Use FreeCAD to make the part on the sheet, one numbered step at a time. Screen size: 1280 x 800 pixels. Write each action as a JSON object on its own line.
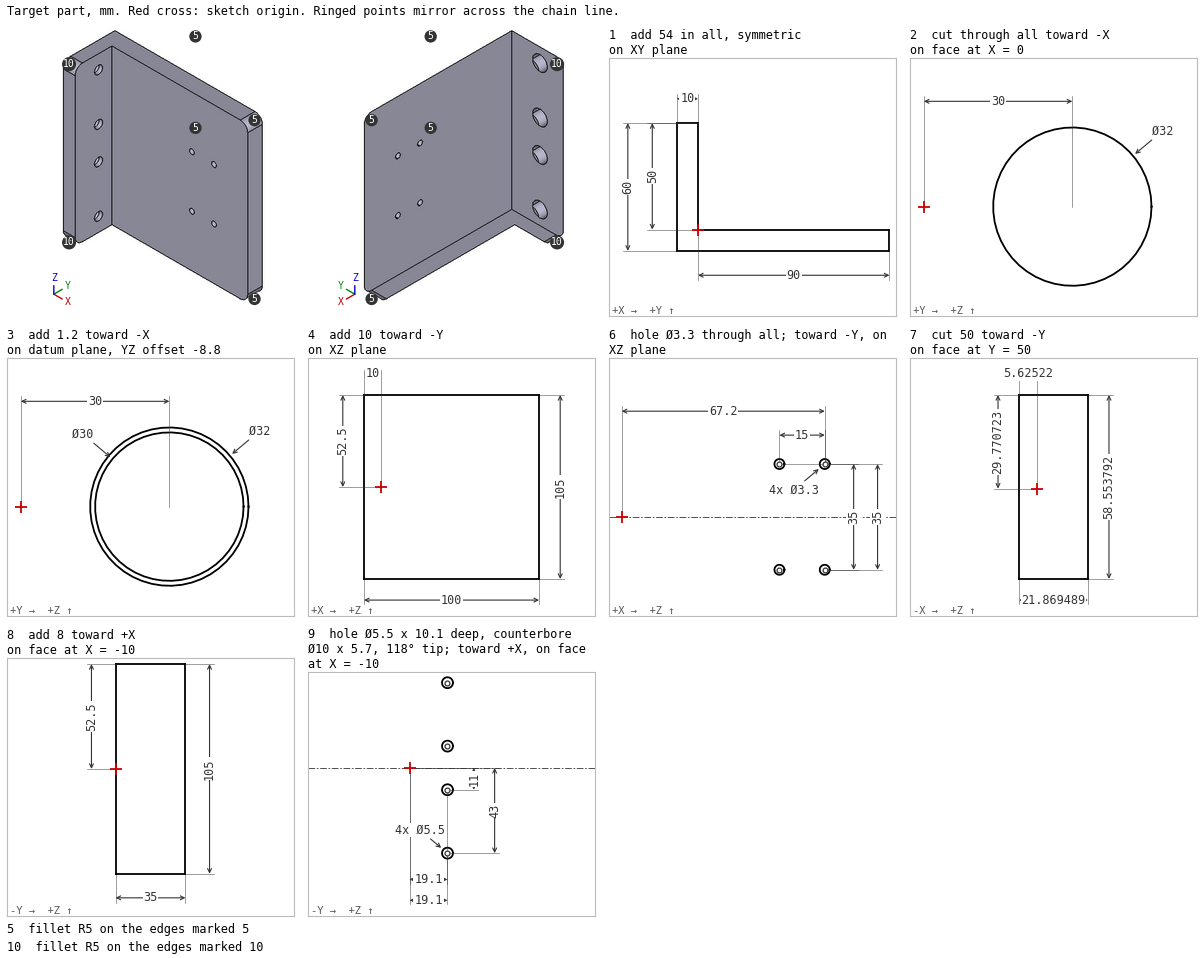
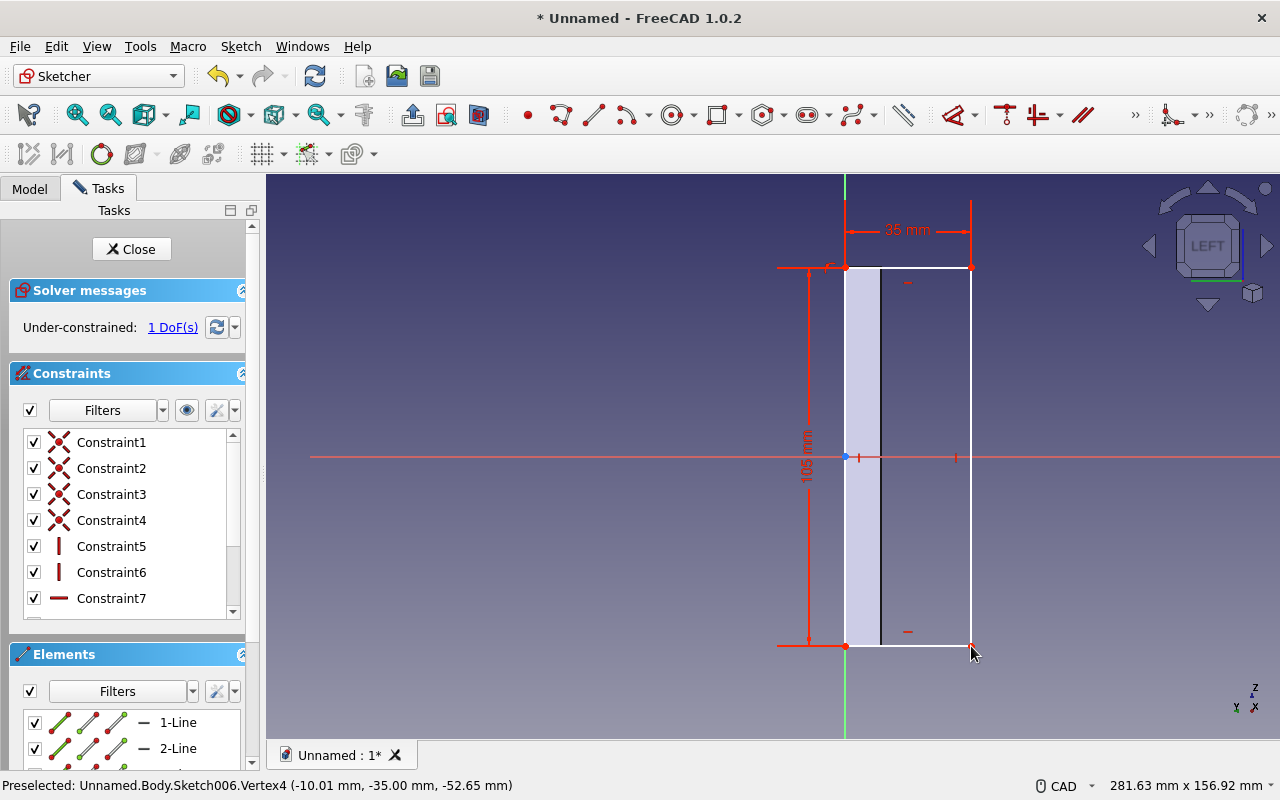
{"action": "left_click", "coordinate": [952, 116]}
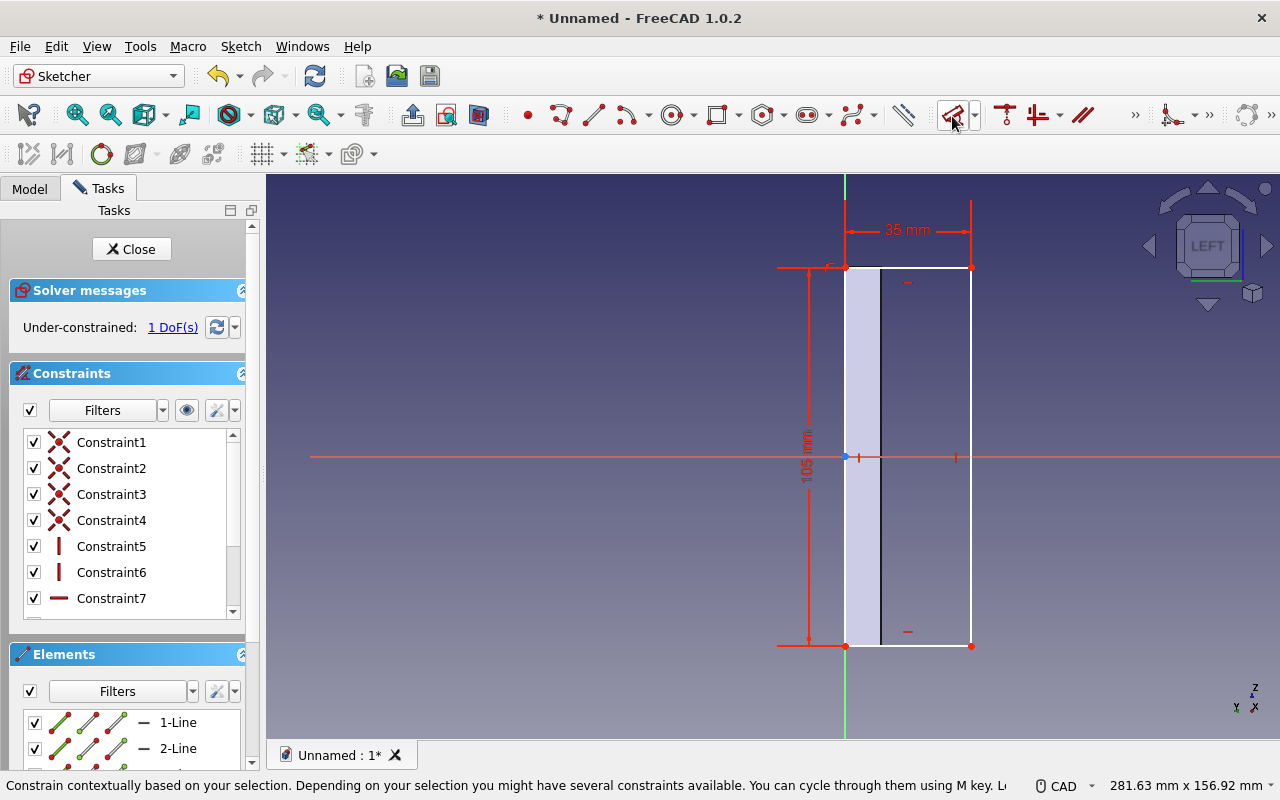
{"action": "left_click", "coordinate": [845, 268]}
{"action": "left_click", "coordinate": [811, 362]}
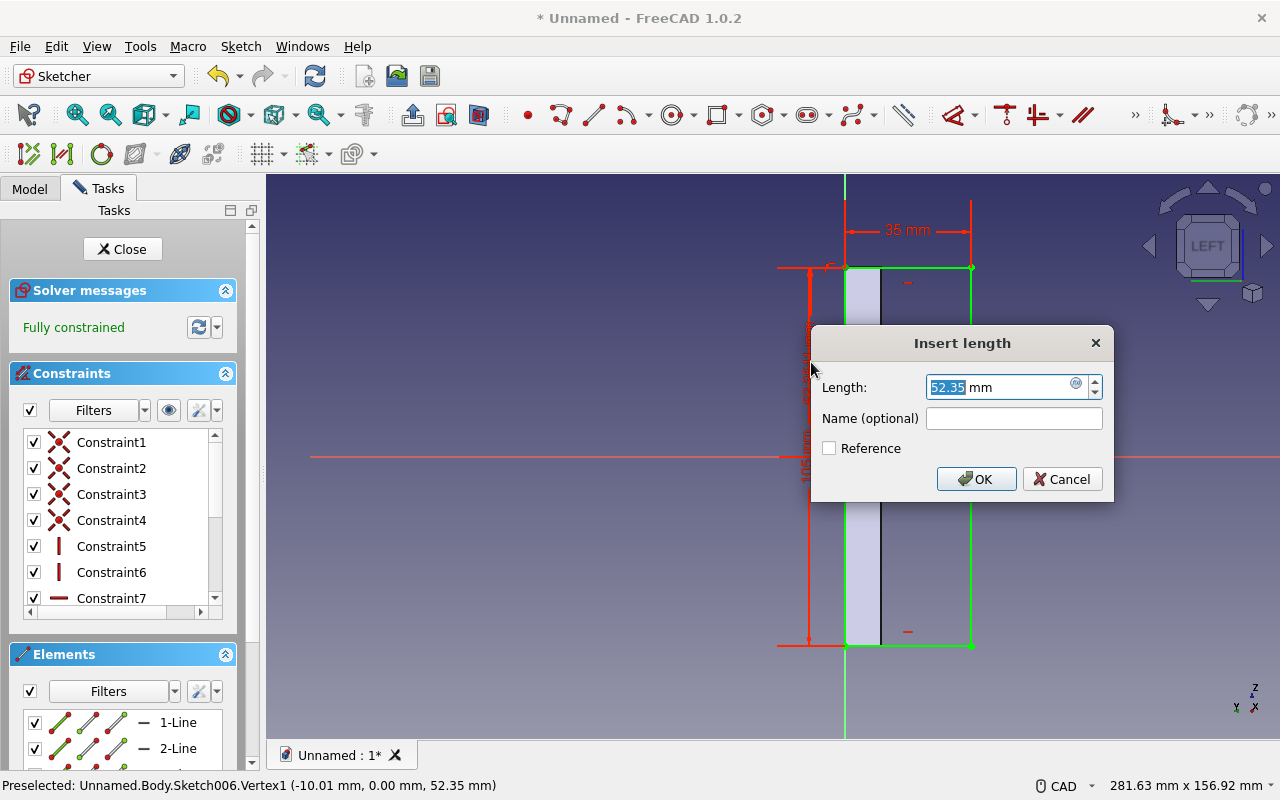
{"action": "type", "text": "52.5"}
{"action": "key", "text": "Return"}
{"action": "key", "text": "Escape"}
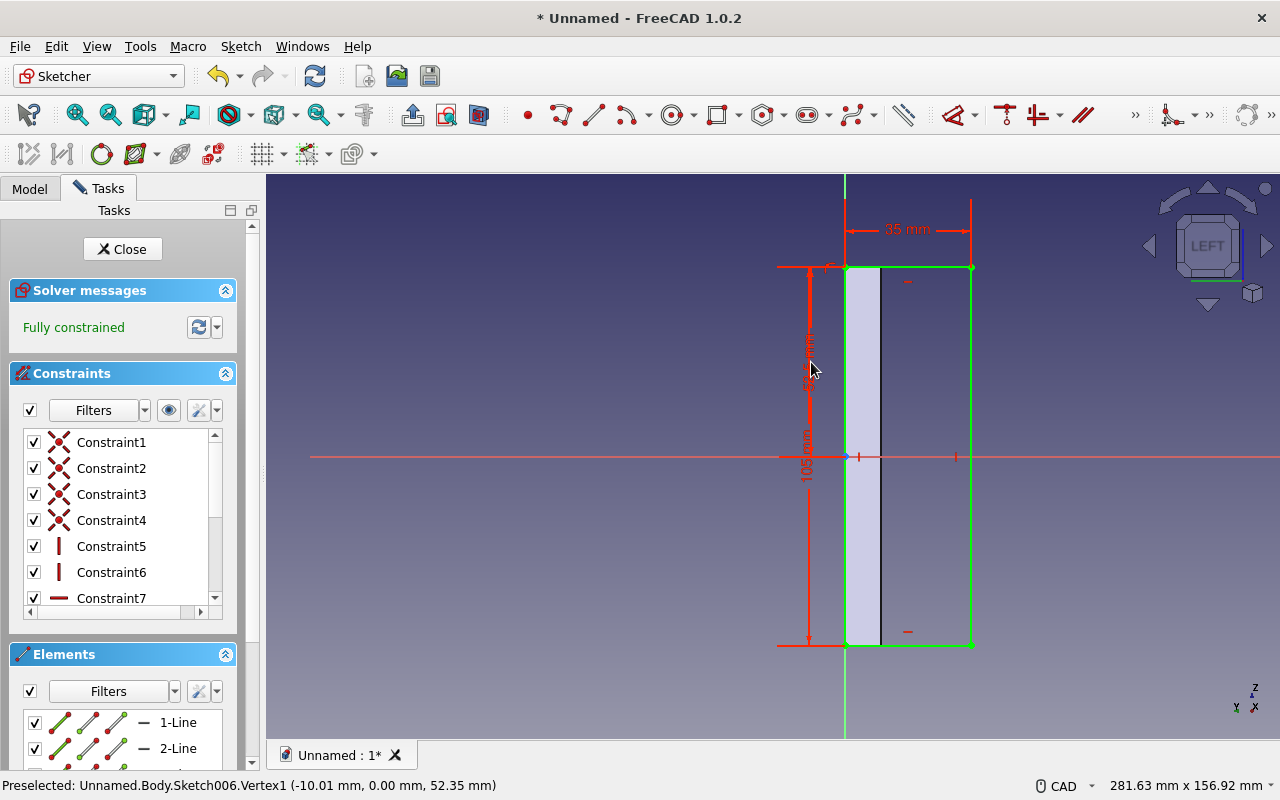
{"action": "left_click", "coordinate": [123, 249]}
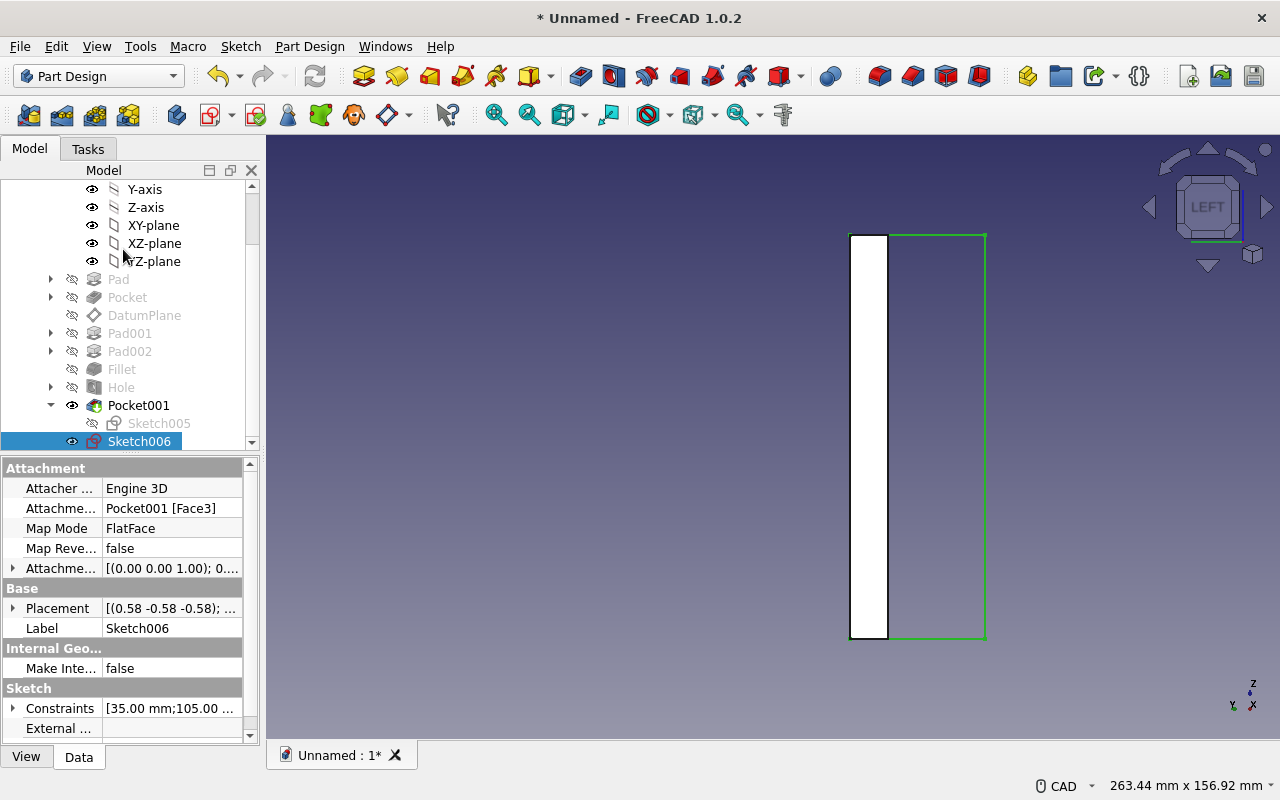
{"action": "left_click", "coordinate": [364, 76]}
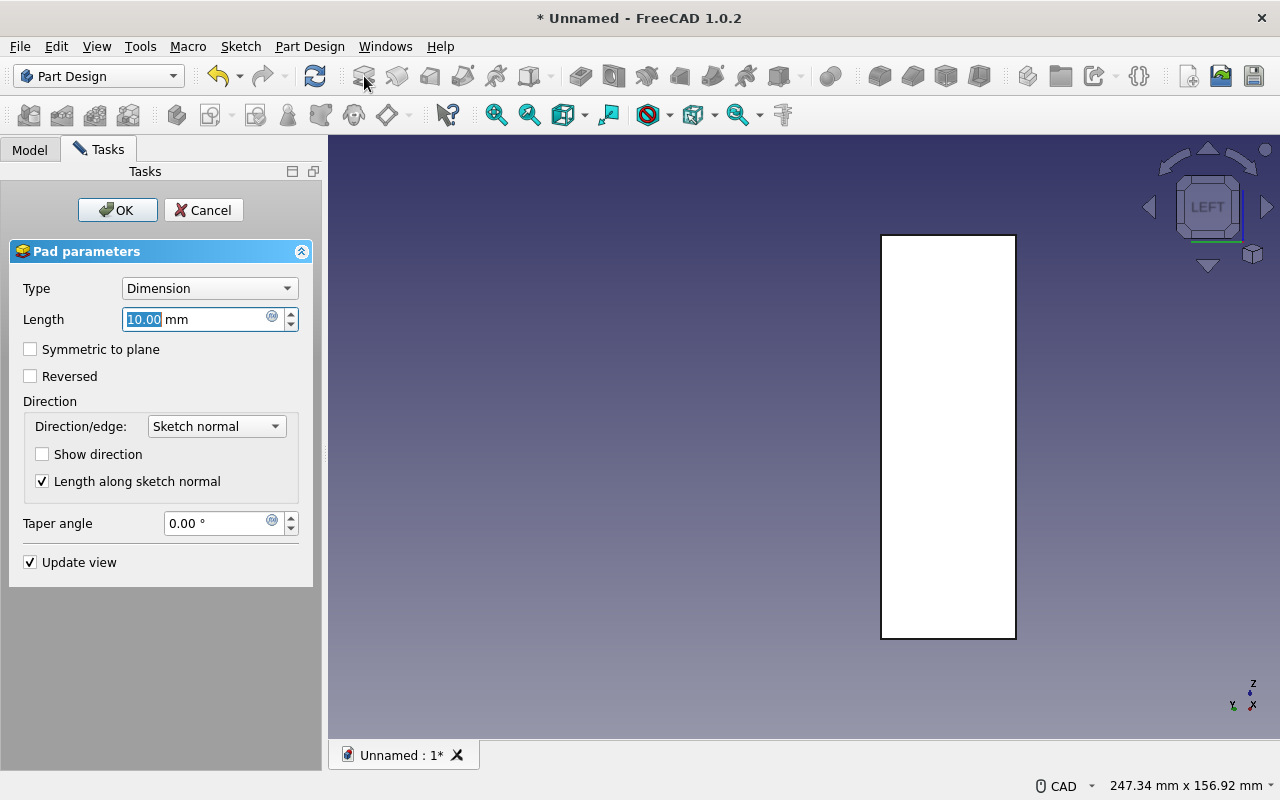
{"action": "type", "text": "8"}
{"action": "key", "text": "Tab"}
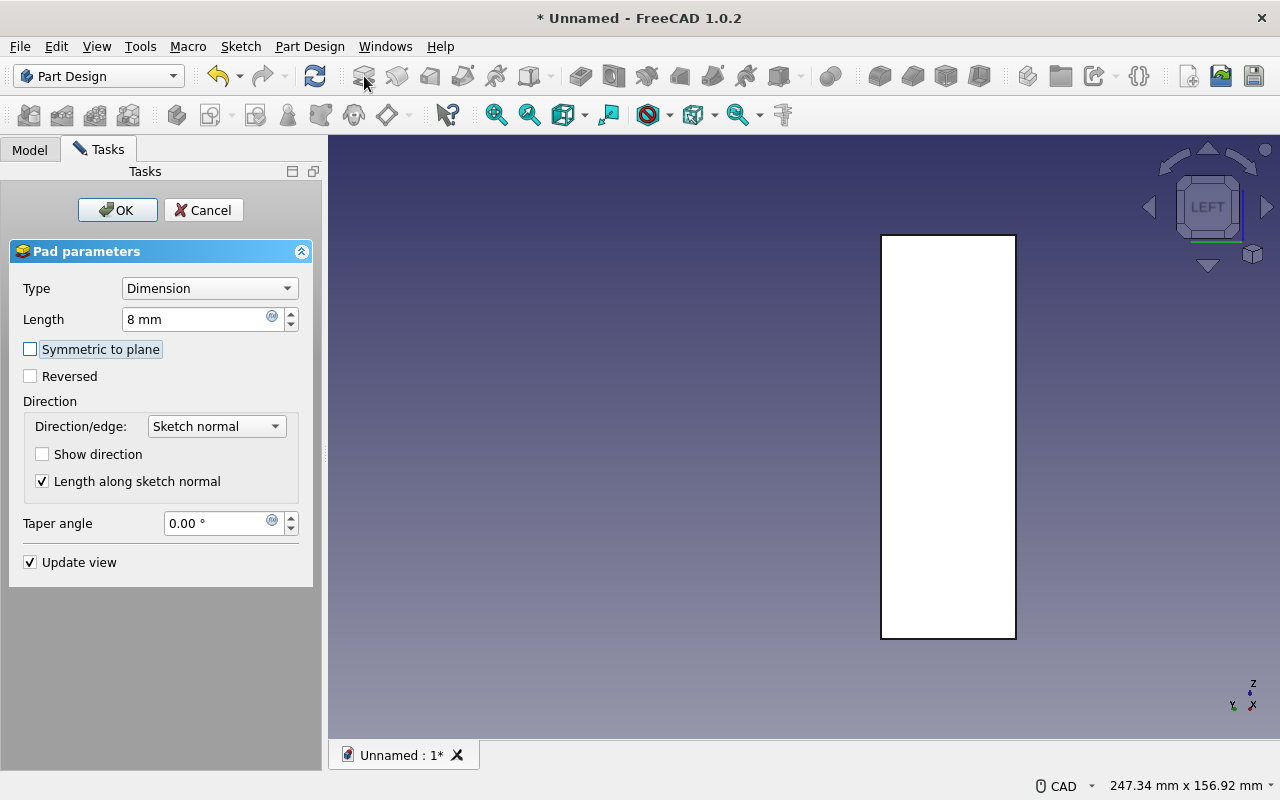
{"action": "left_click", "coordinate": [31, 376]}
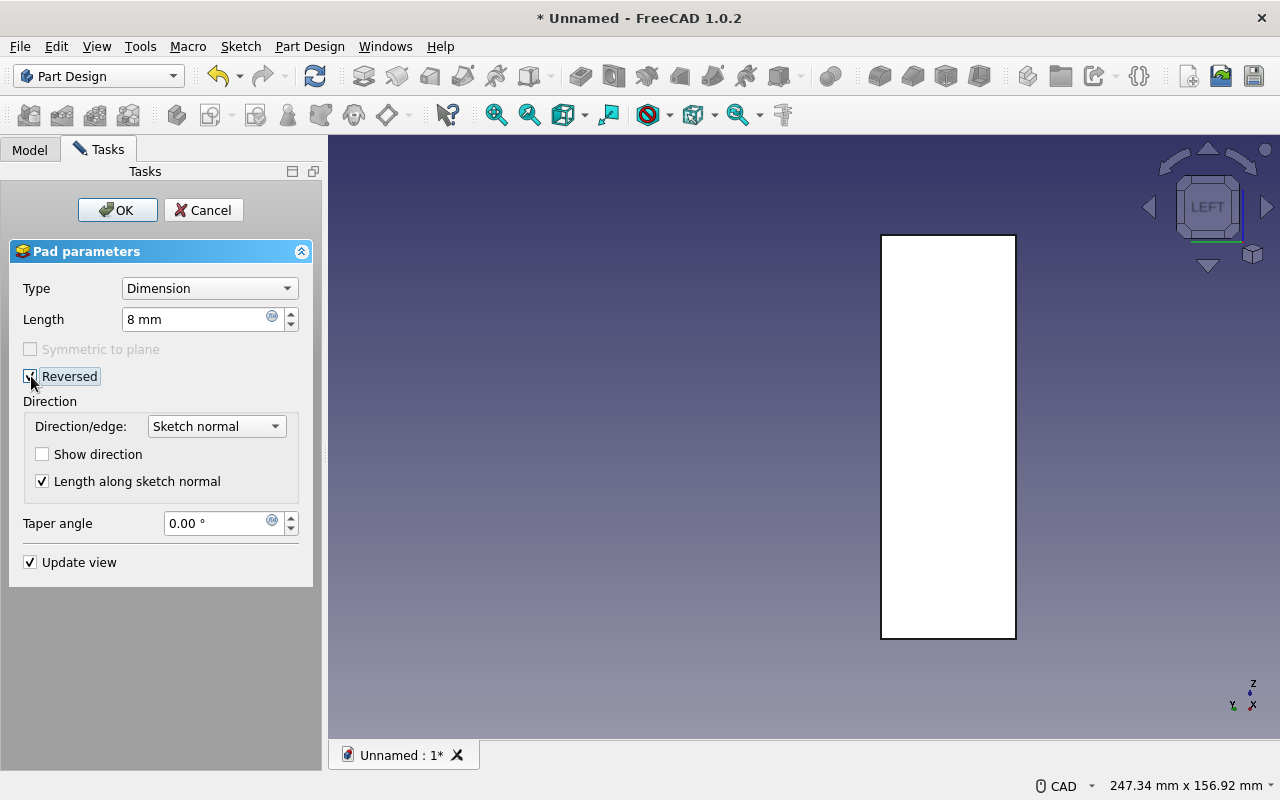
{"action": "left_click", "coordinate": [118, 210]}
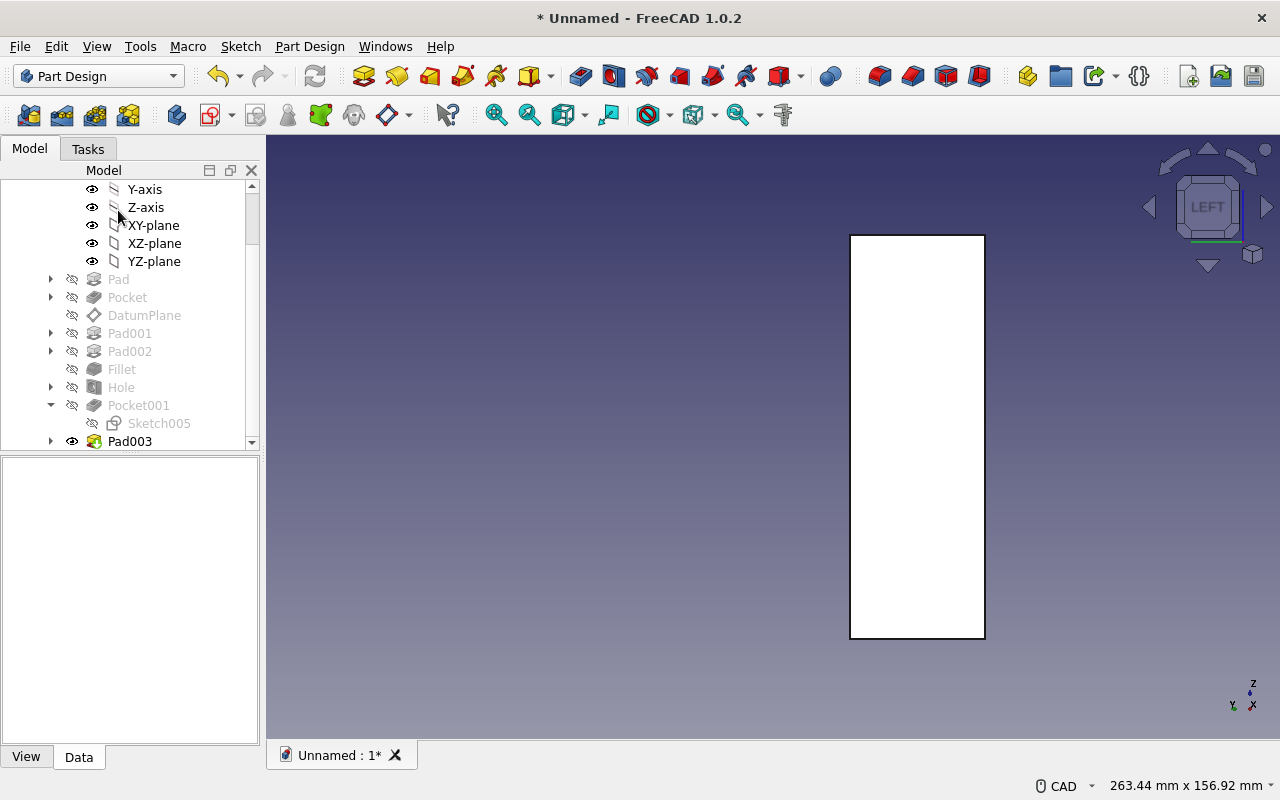
{"action": "left_click", "coordinate": [917, 321]}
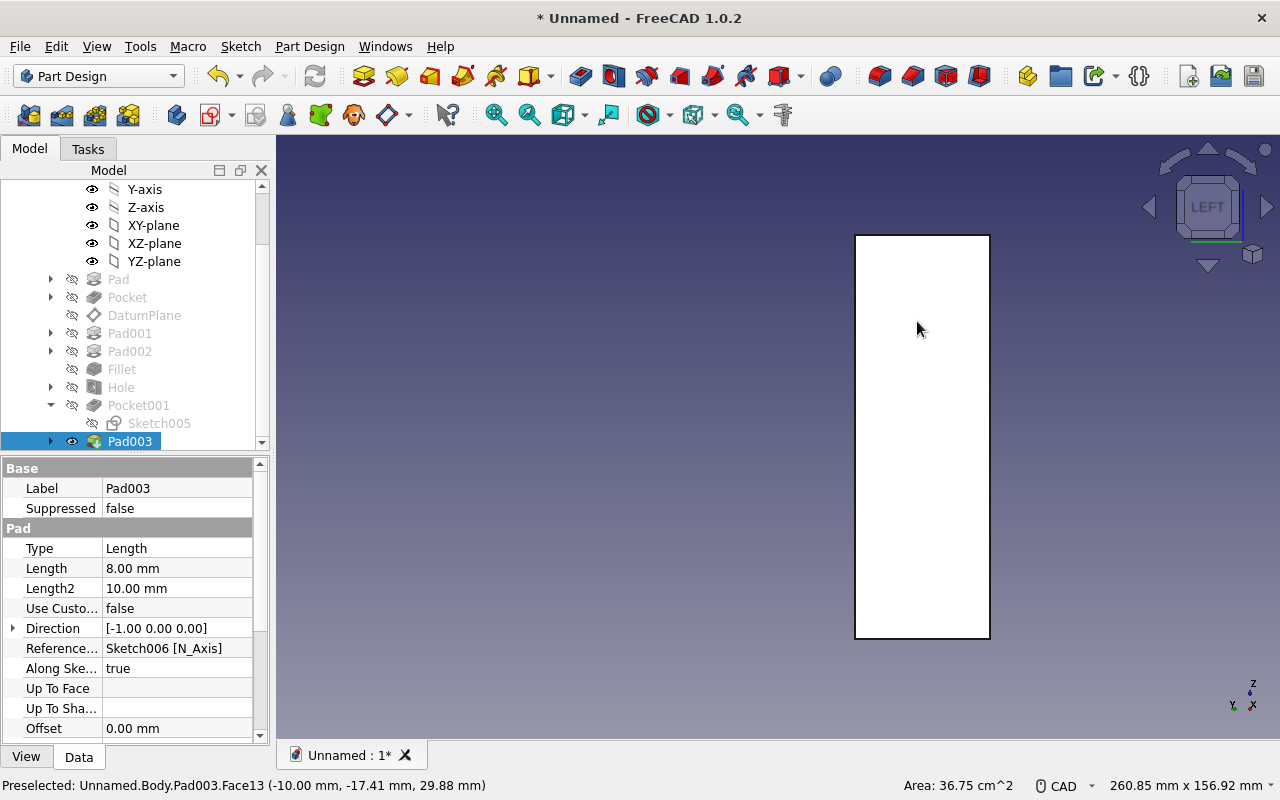
{"action": "left_click", "coordinate": [210, 116]}